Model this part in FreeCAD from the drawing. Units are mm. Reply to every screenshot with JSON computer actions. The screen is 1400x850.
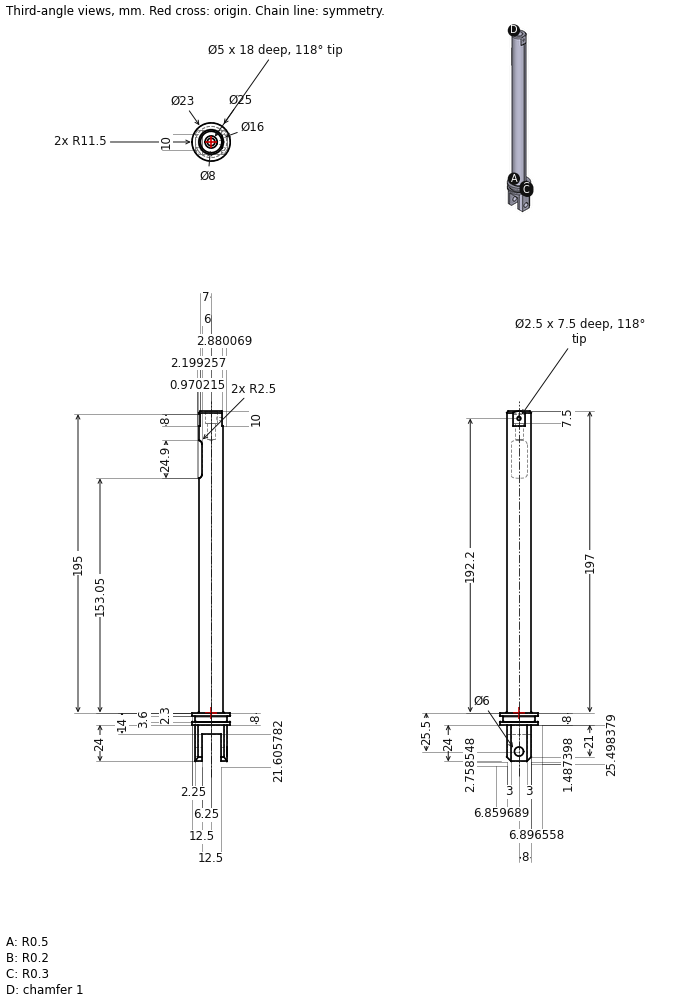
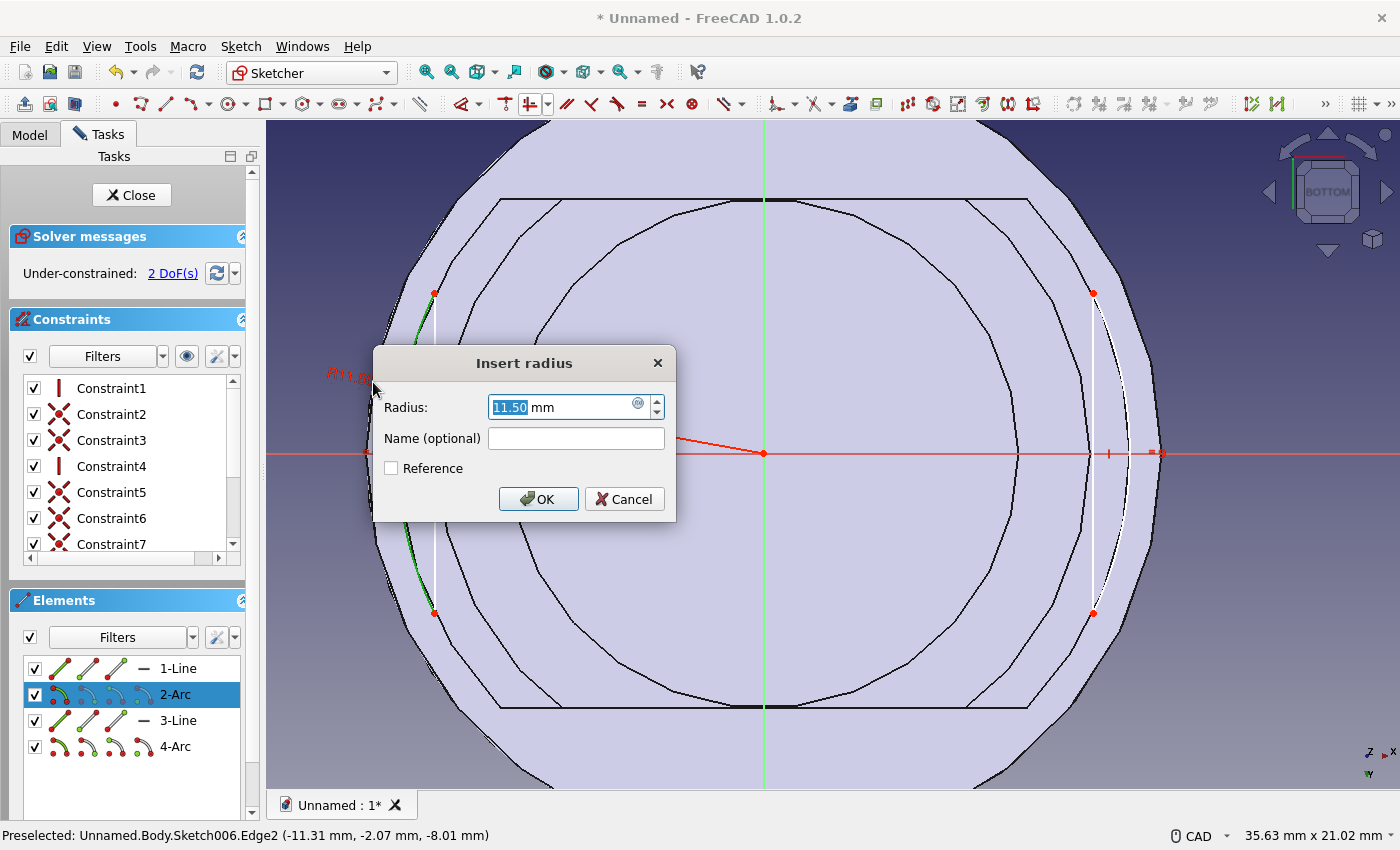
{"action": "type", "text": "11.5"}
{"action": "key", "text": "Return"}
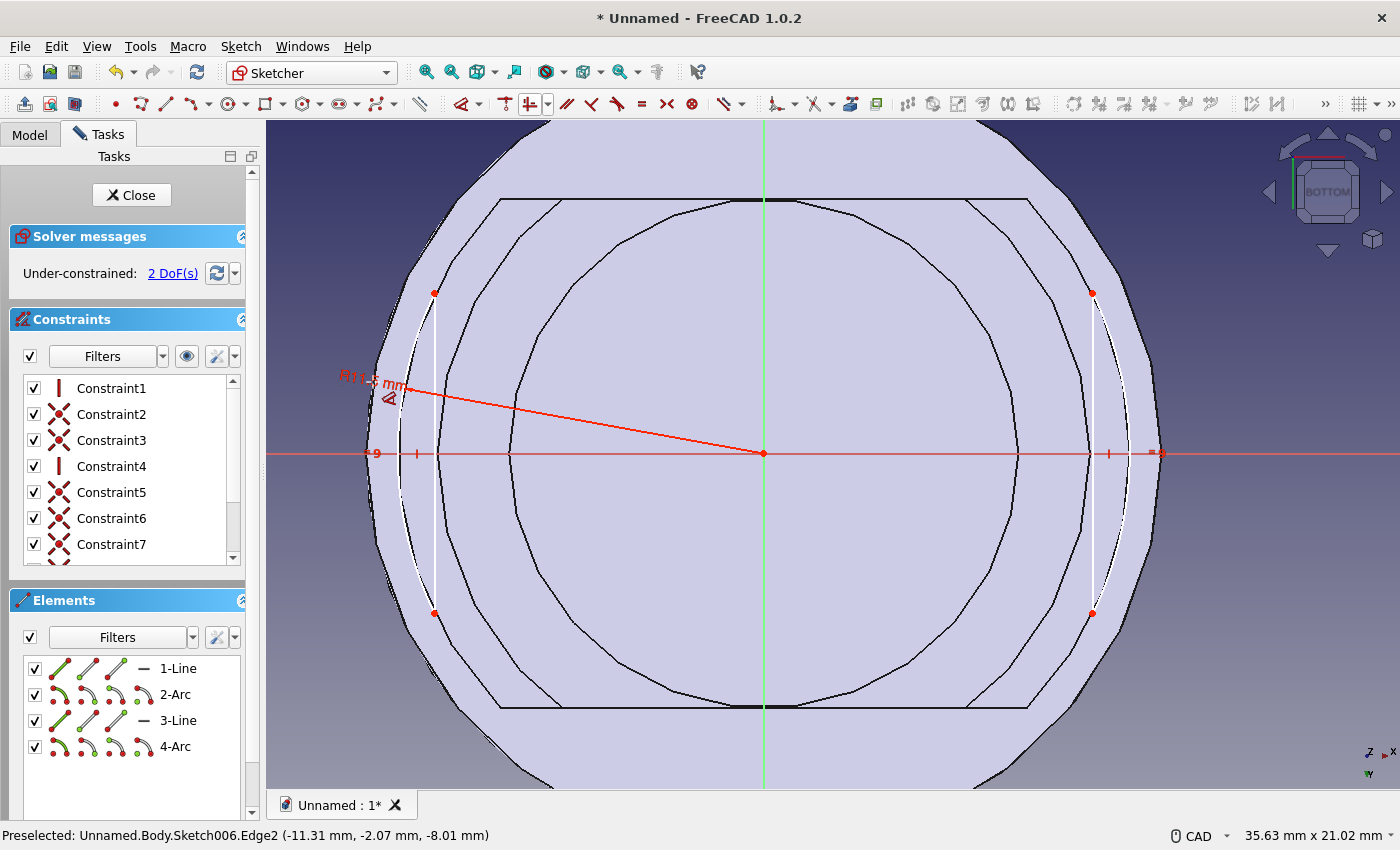
{"action": "left_click", "coordinate": [435, 518]}
{"action": "left_click", "coordinate": [401, 342]}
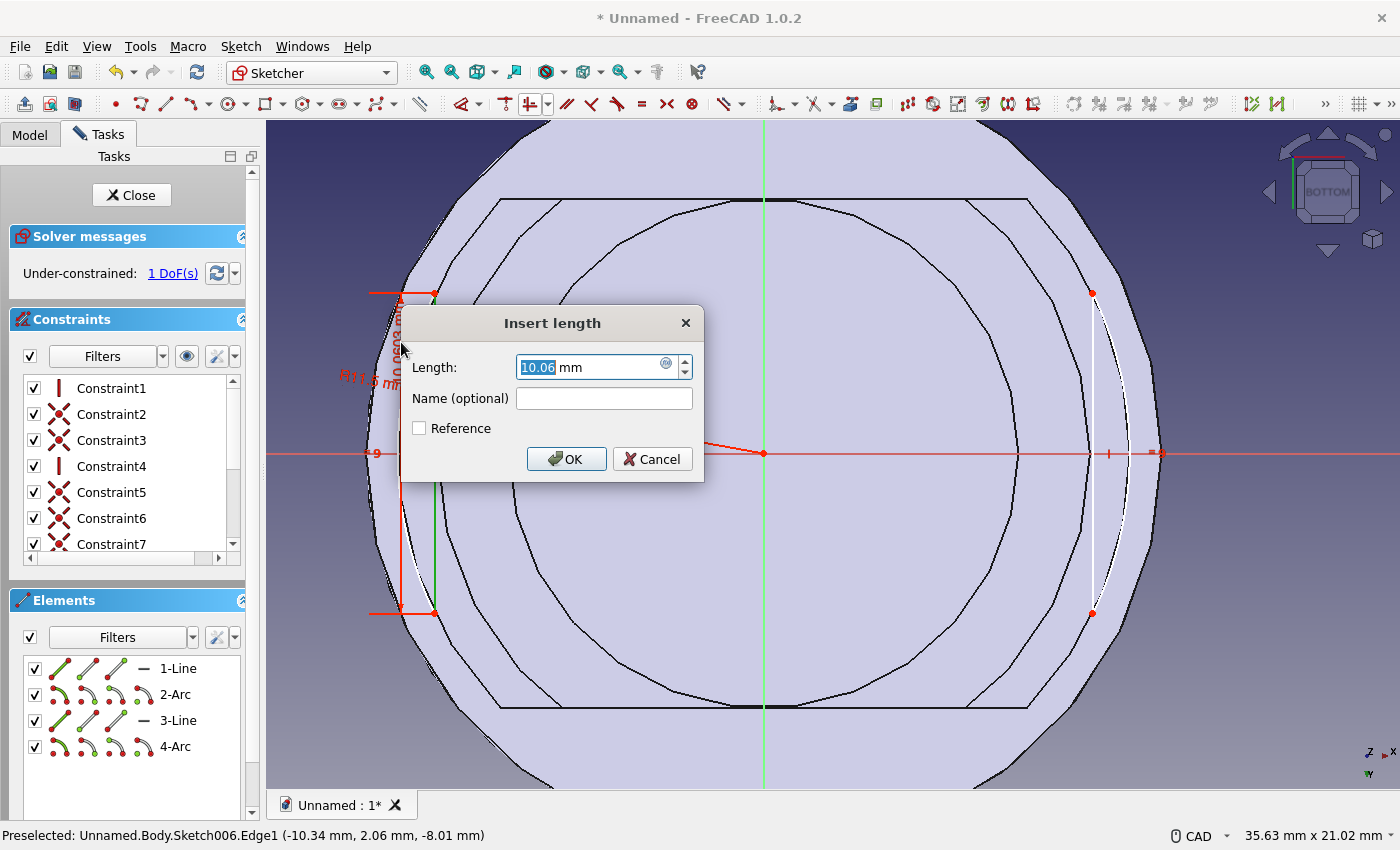
{"action": "type", "text": "10"}
{"action": "key", "text": "Return"}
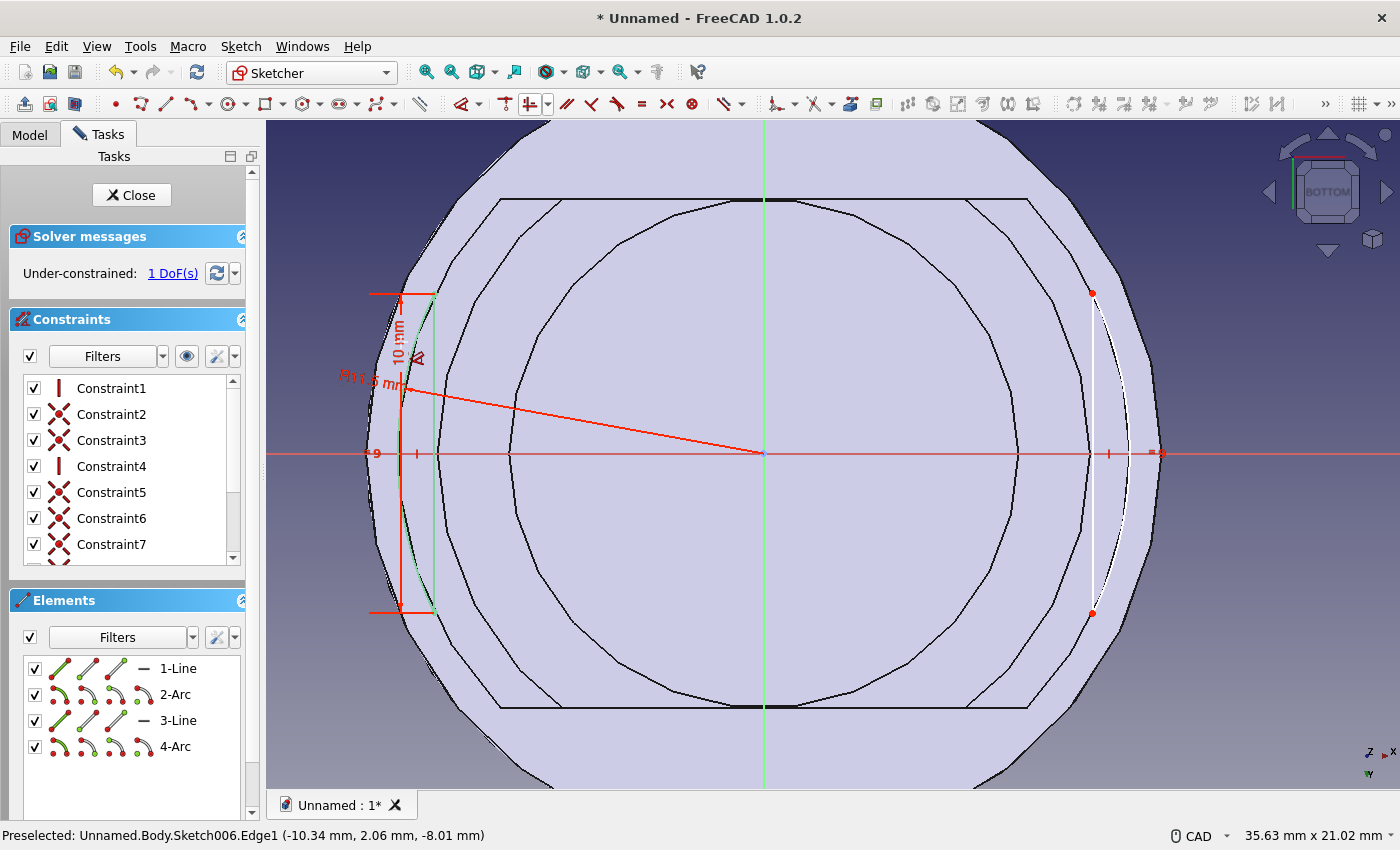
{"action": "left_click", "coordinate": [1093, 390]}
{"action": "left_click", "coordinate": [1127, 342]}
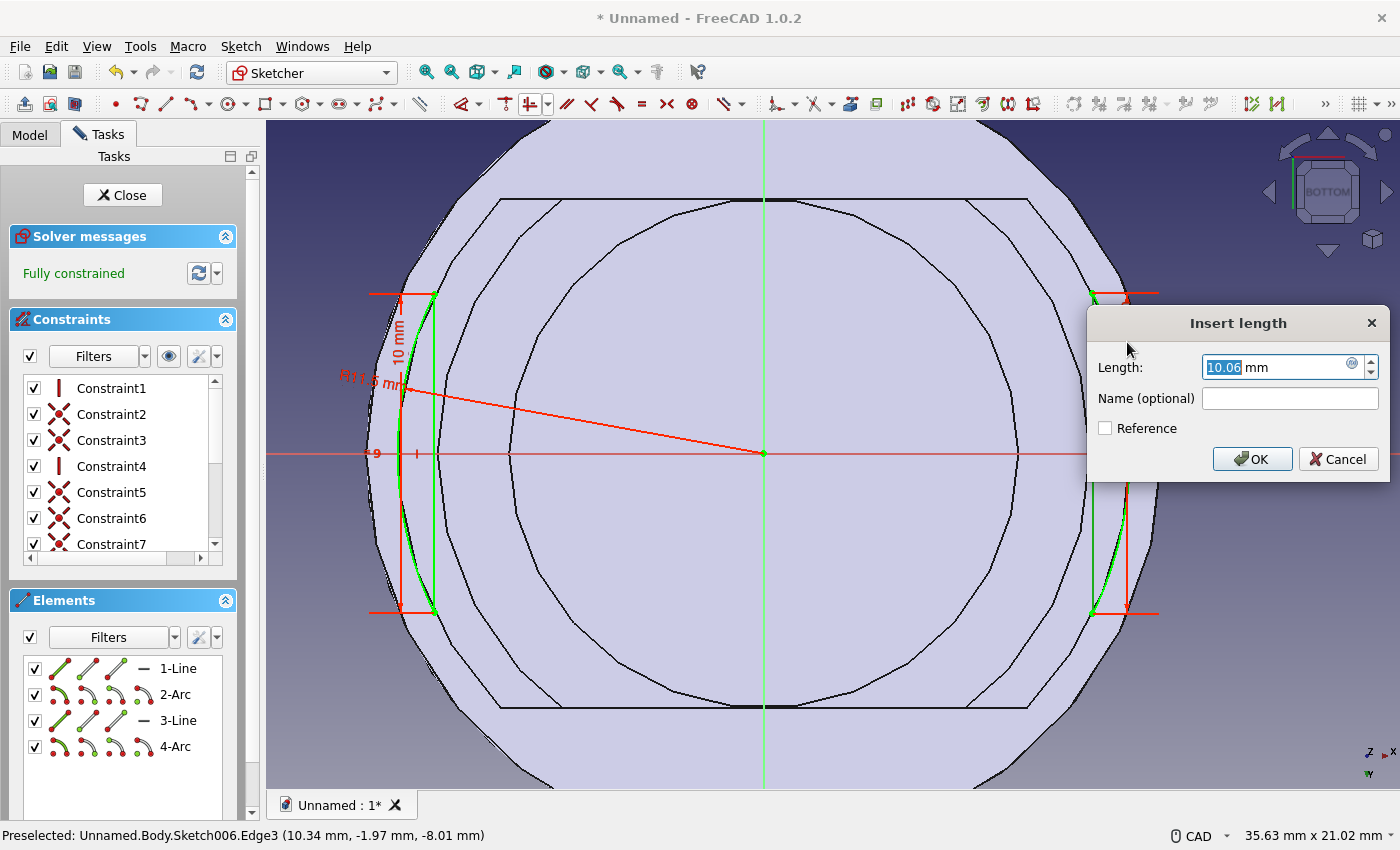
{"action": "type", "text": "10"}
{"action": "key", "text": "Return"}
{"action": "key", "text": "Escape"}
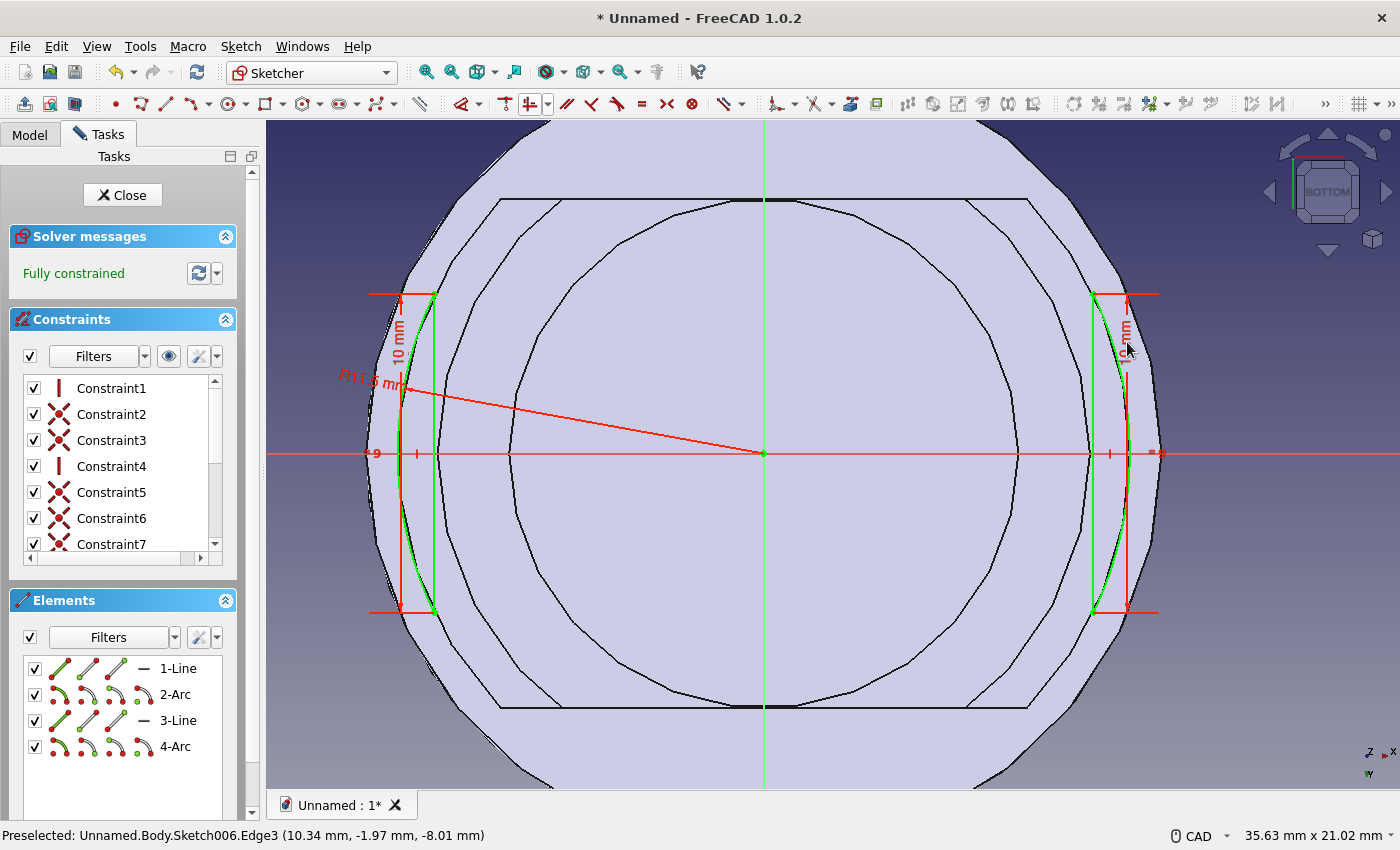
{"action": "left_click", "coordinate": [123, 195]}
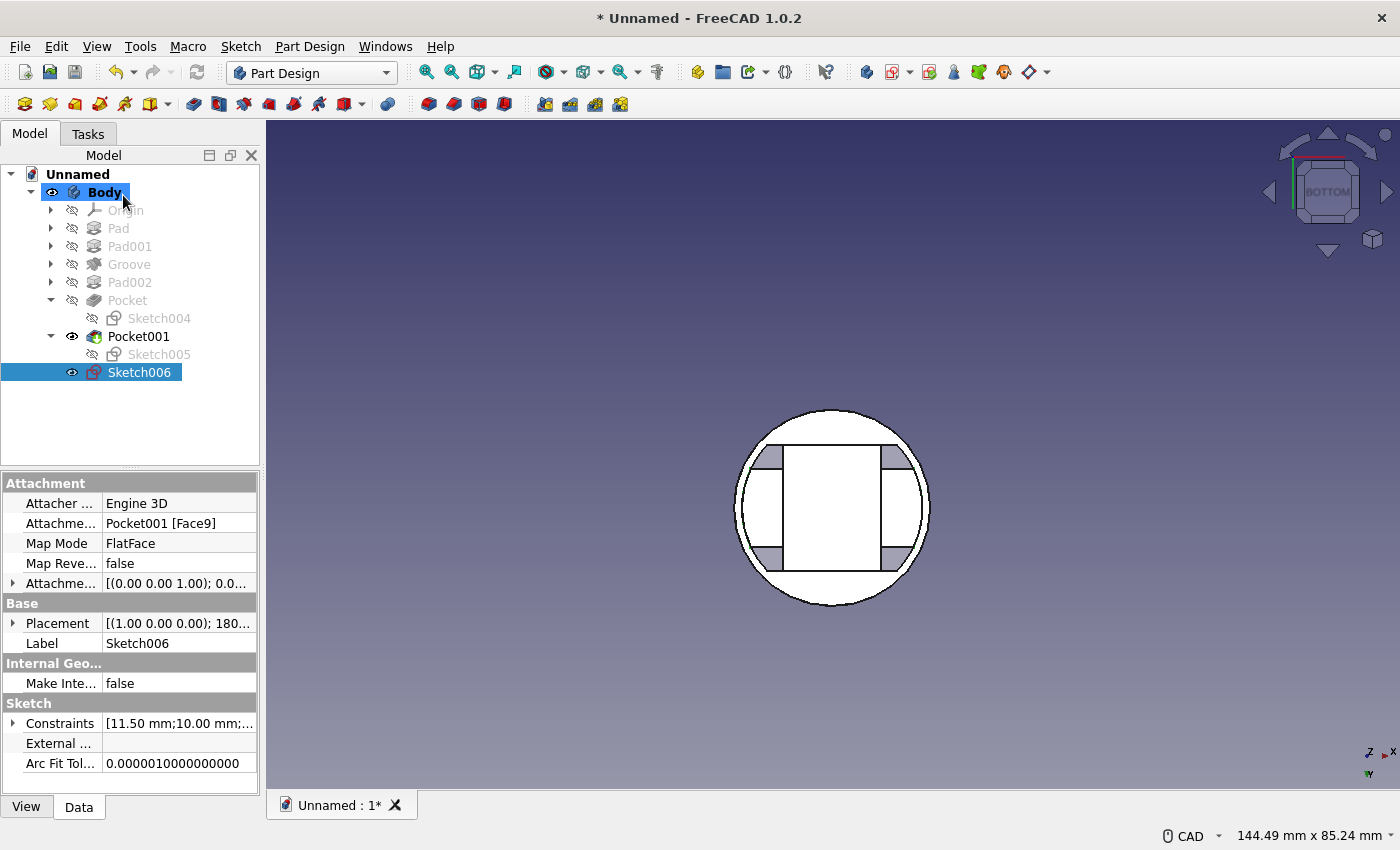
{"action": "left_click", "coordinate": [194, 104]}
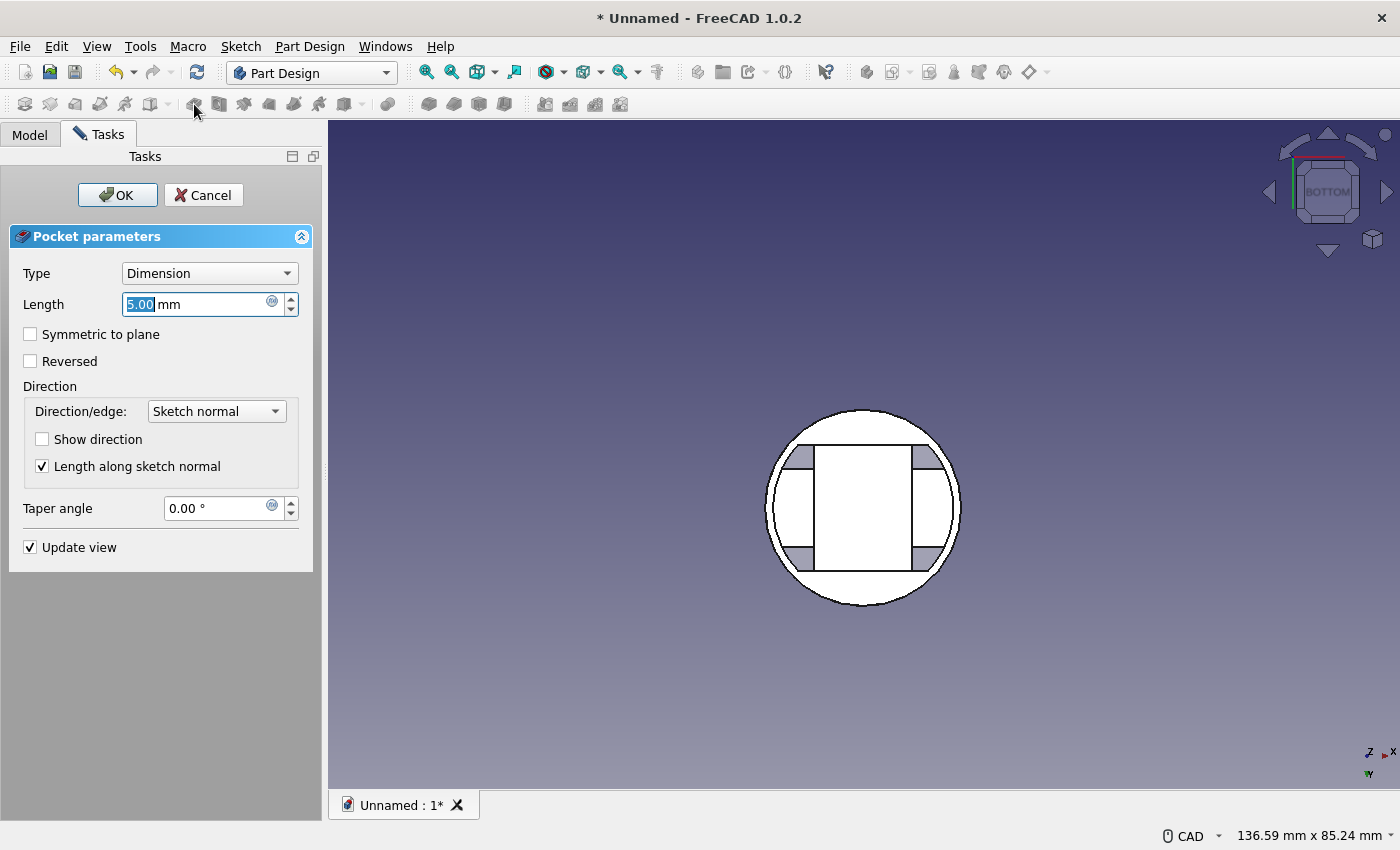
{"action": "type", "text": "24"}
{"action": "key", "text": "Tab"}